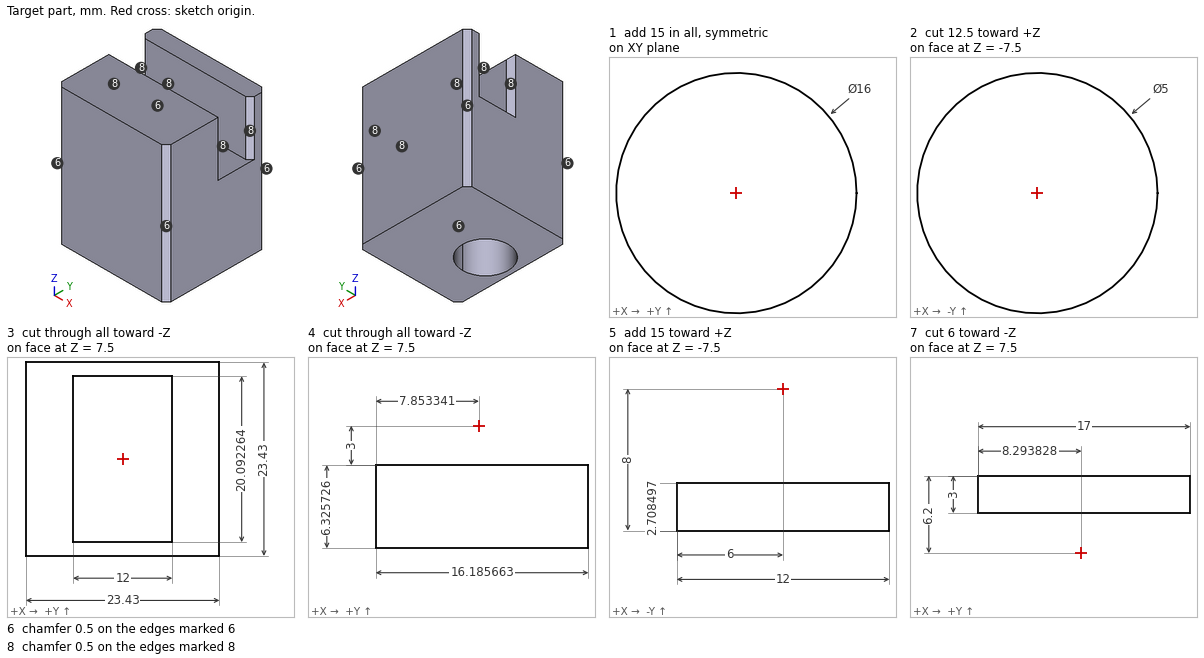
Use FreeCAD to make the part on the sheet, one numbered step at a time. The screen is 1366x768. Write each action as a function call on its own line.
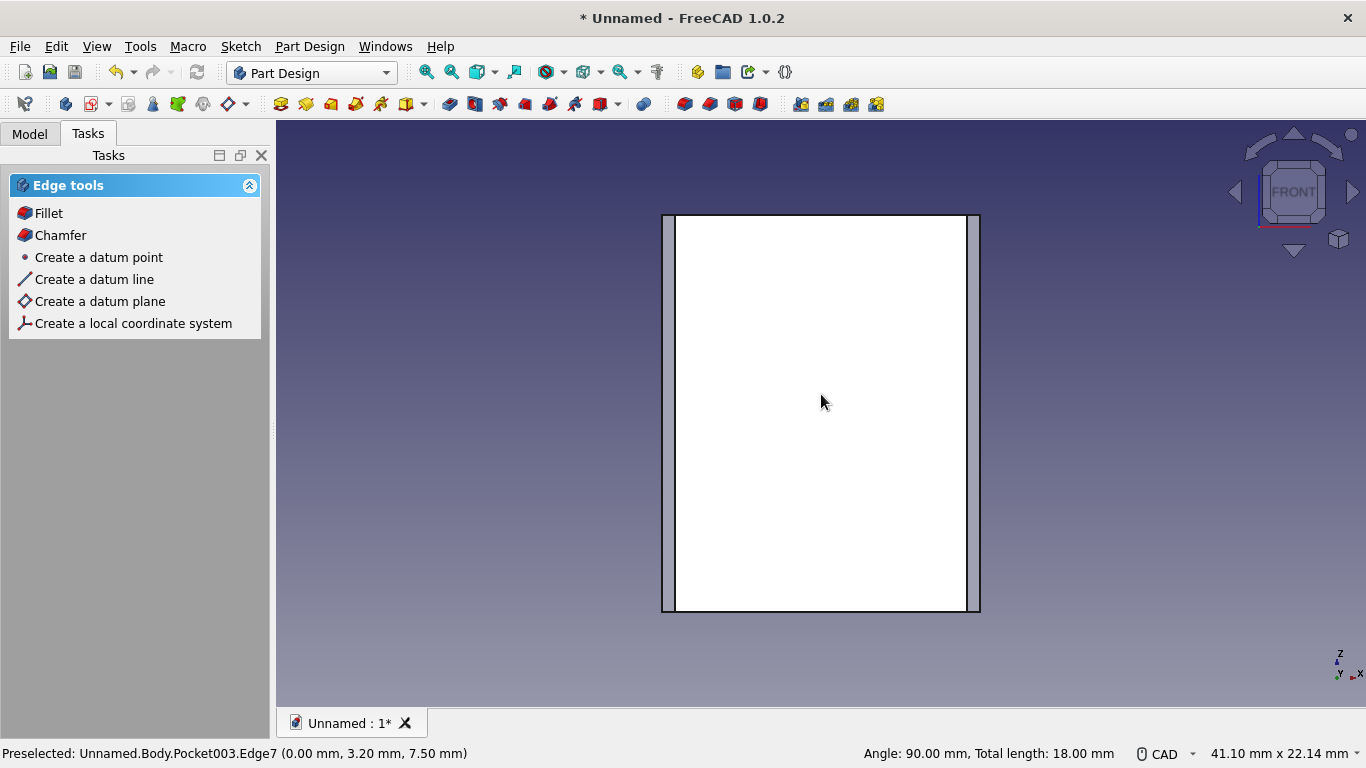
key(3)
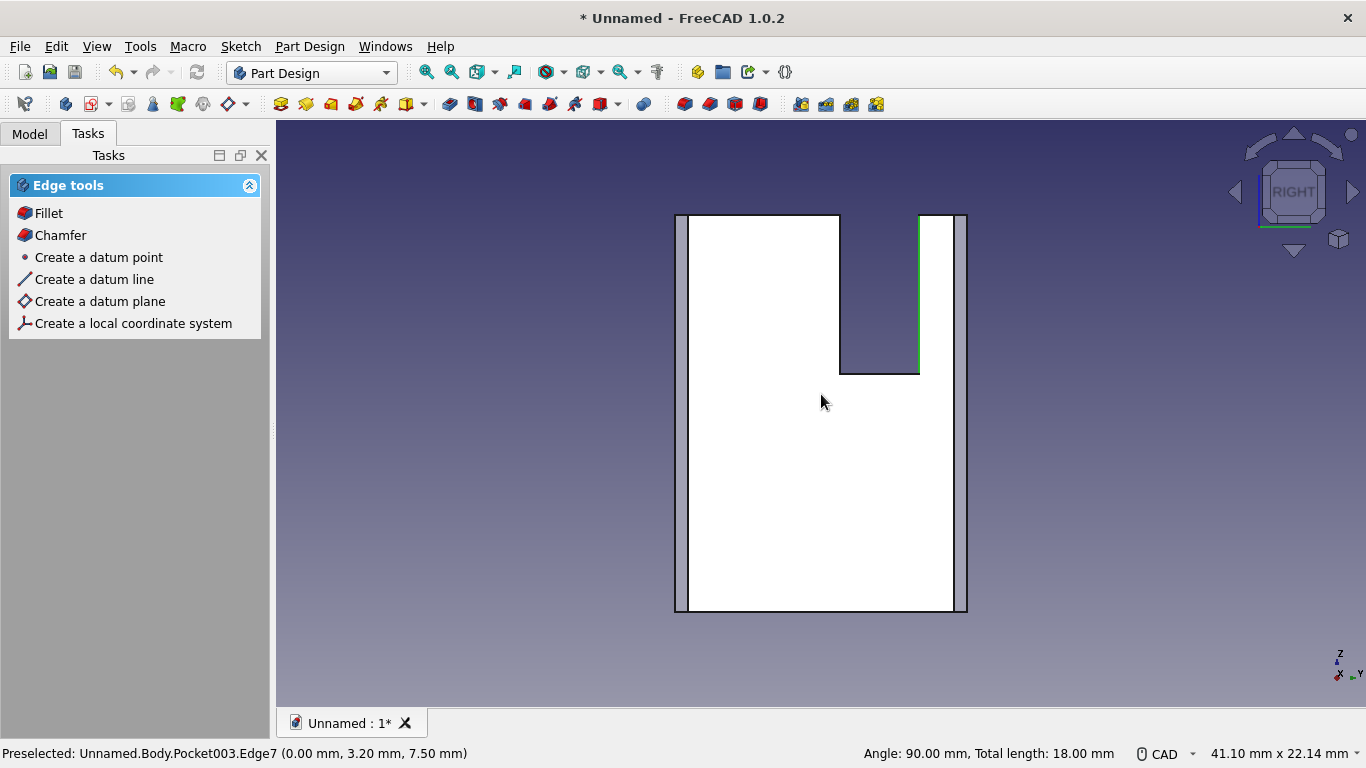
click(840, 293, ctrl)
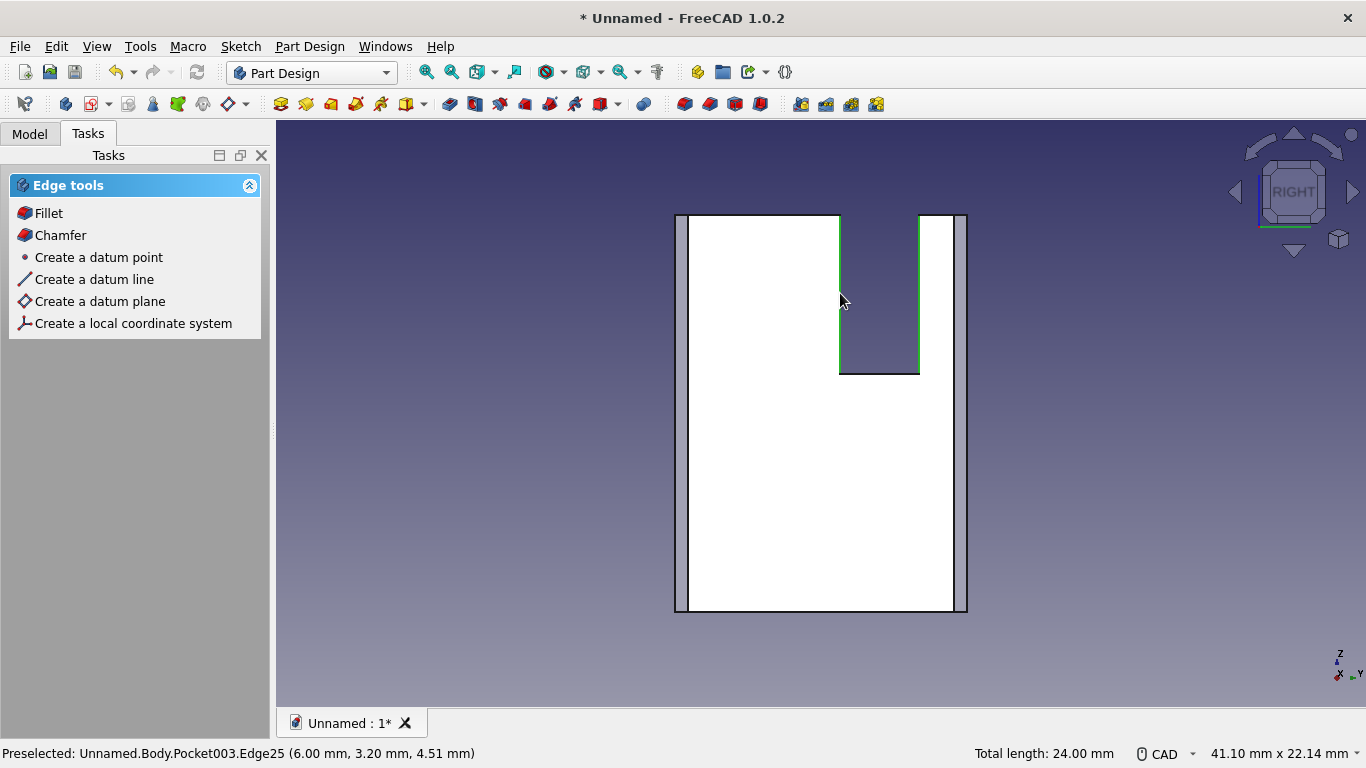
key(5)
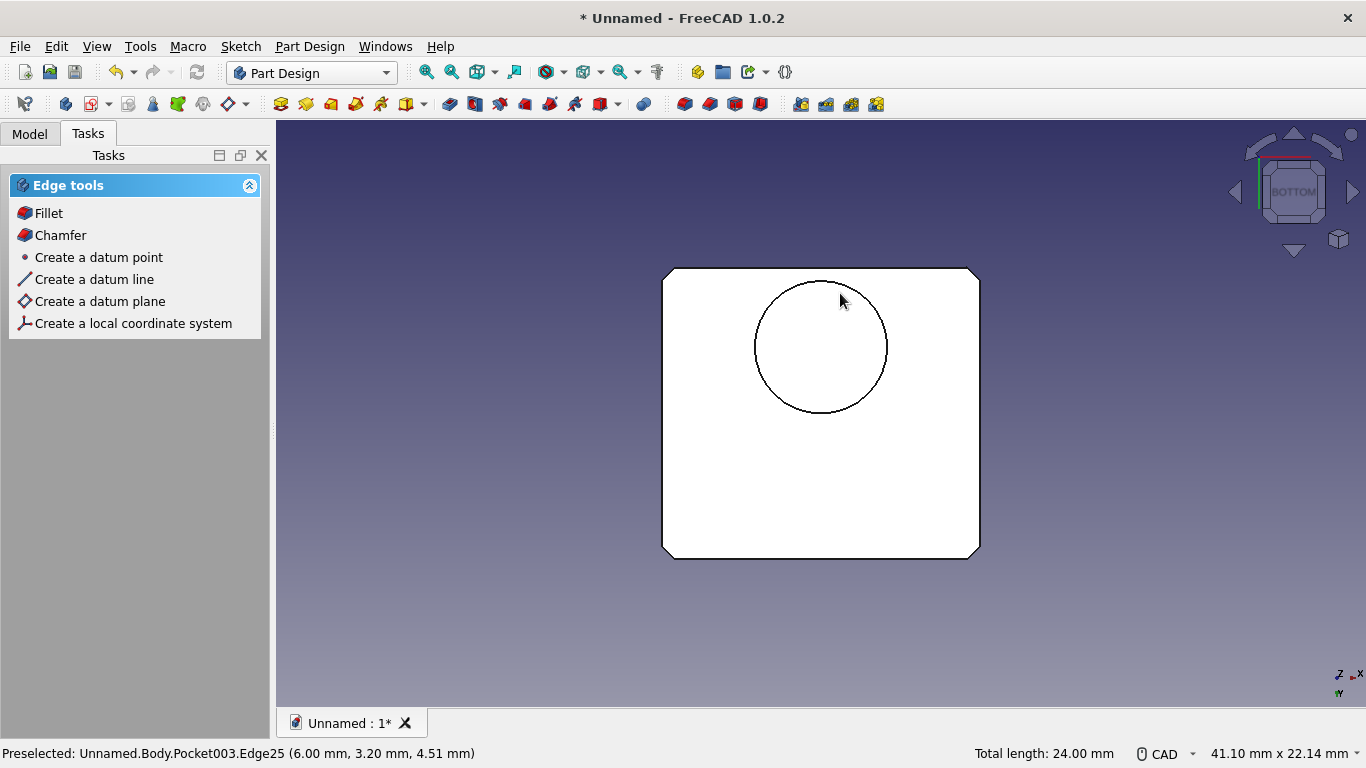
key(4)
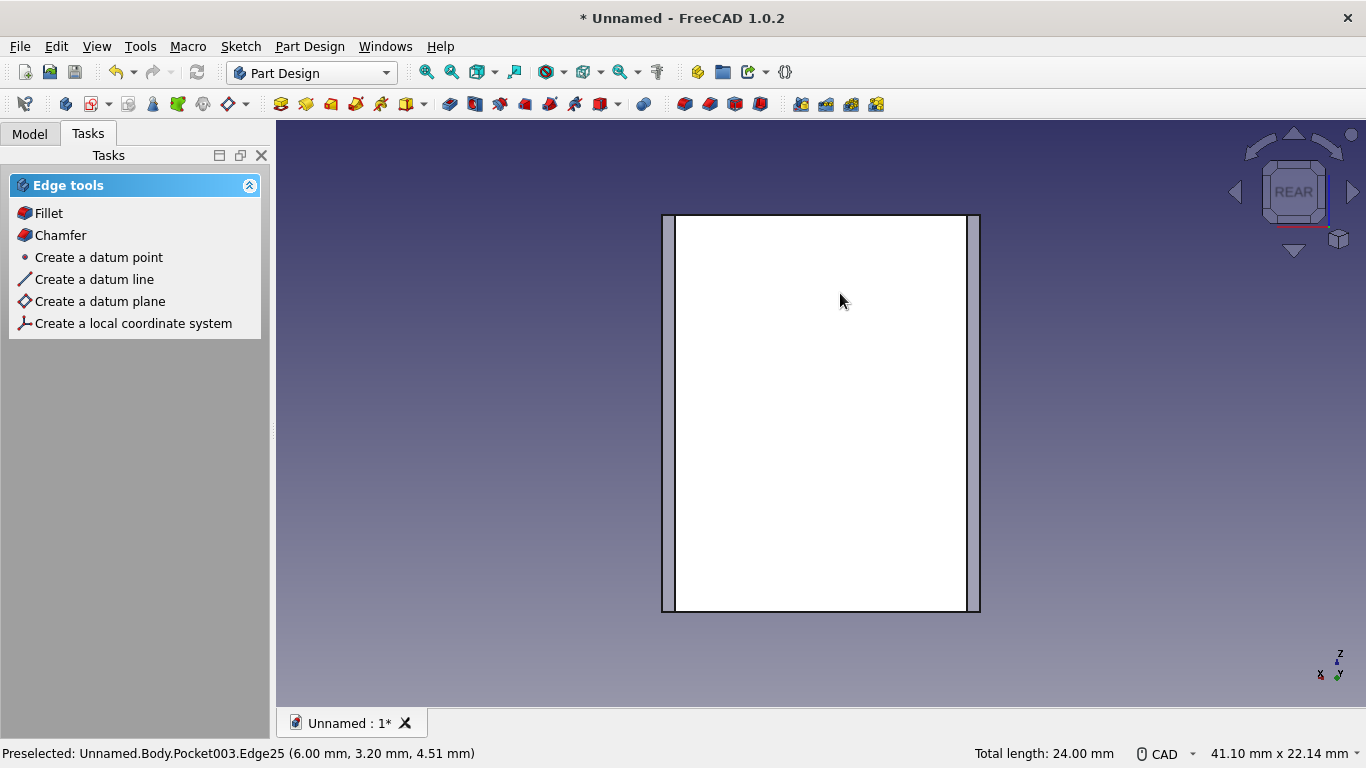
key(6)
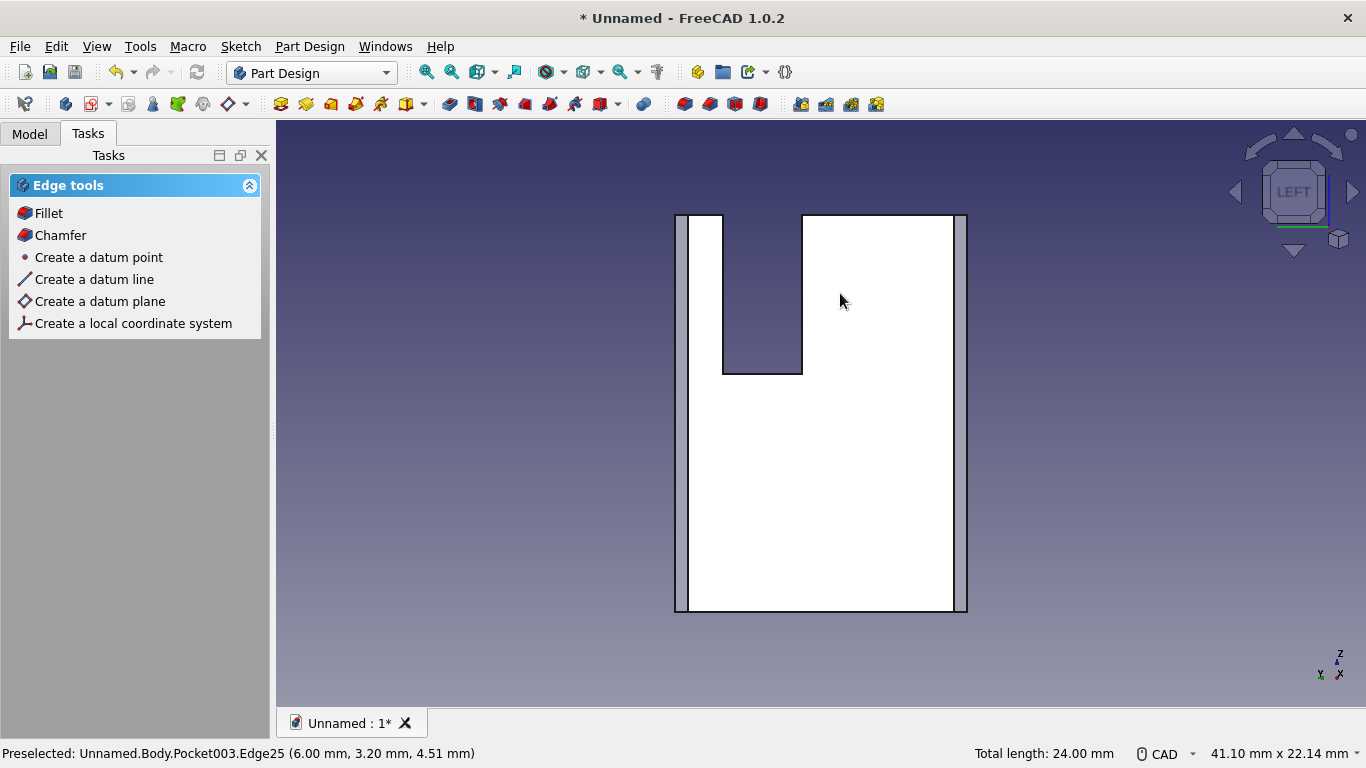
click(723, 293, ctrl)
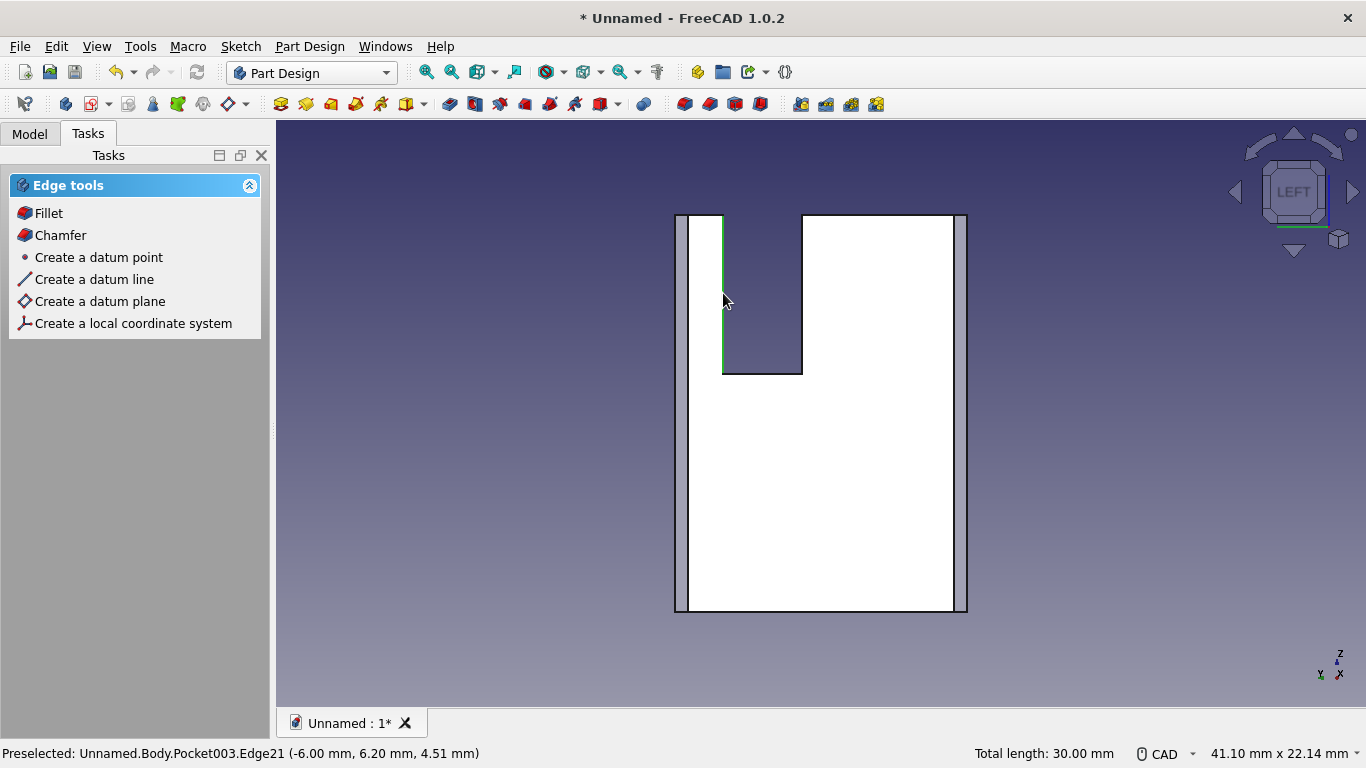
click(802, 293, ctrl)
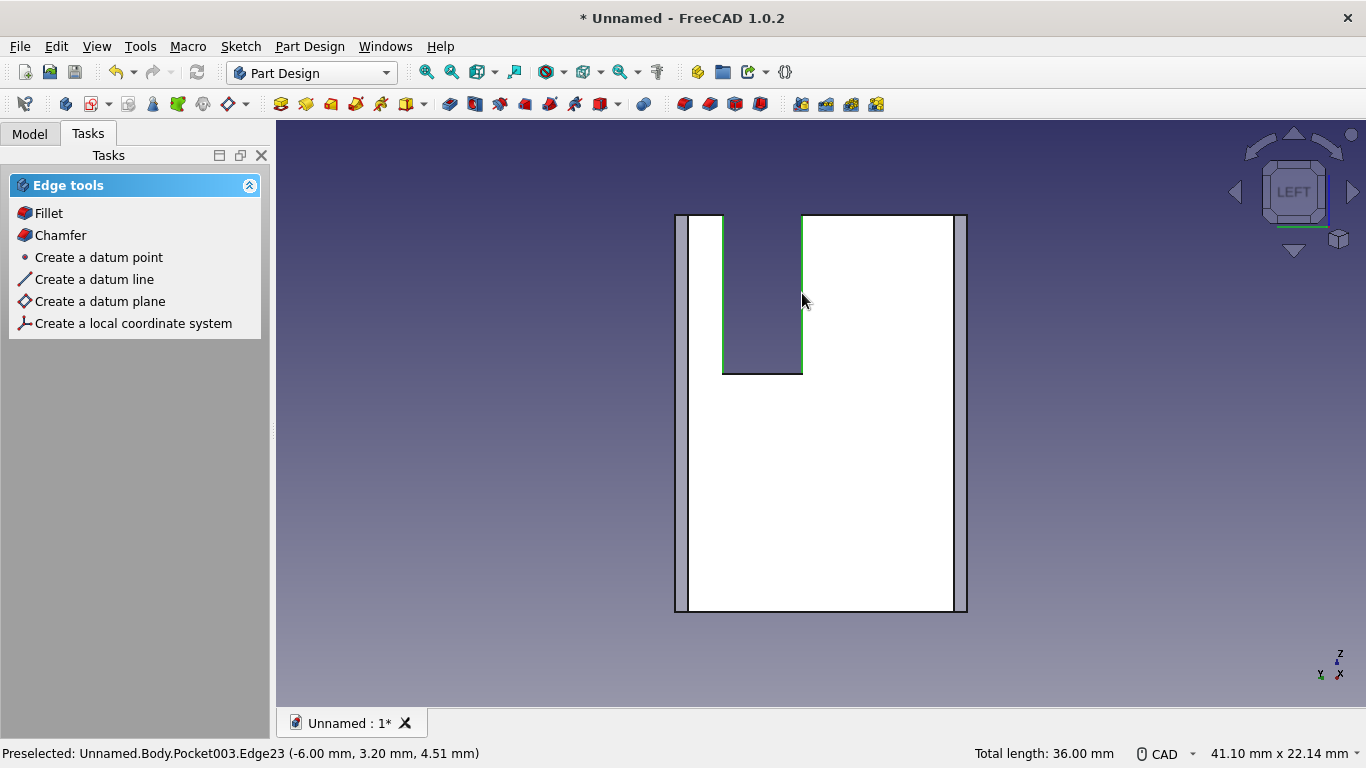
click(710, 104)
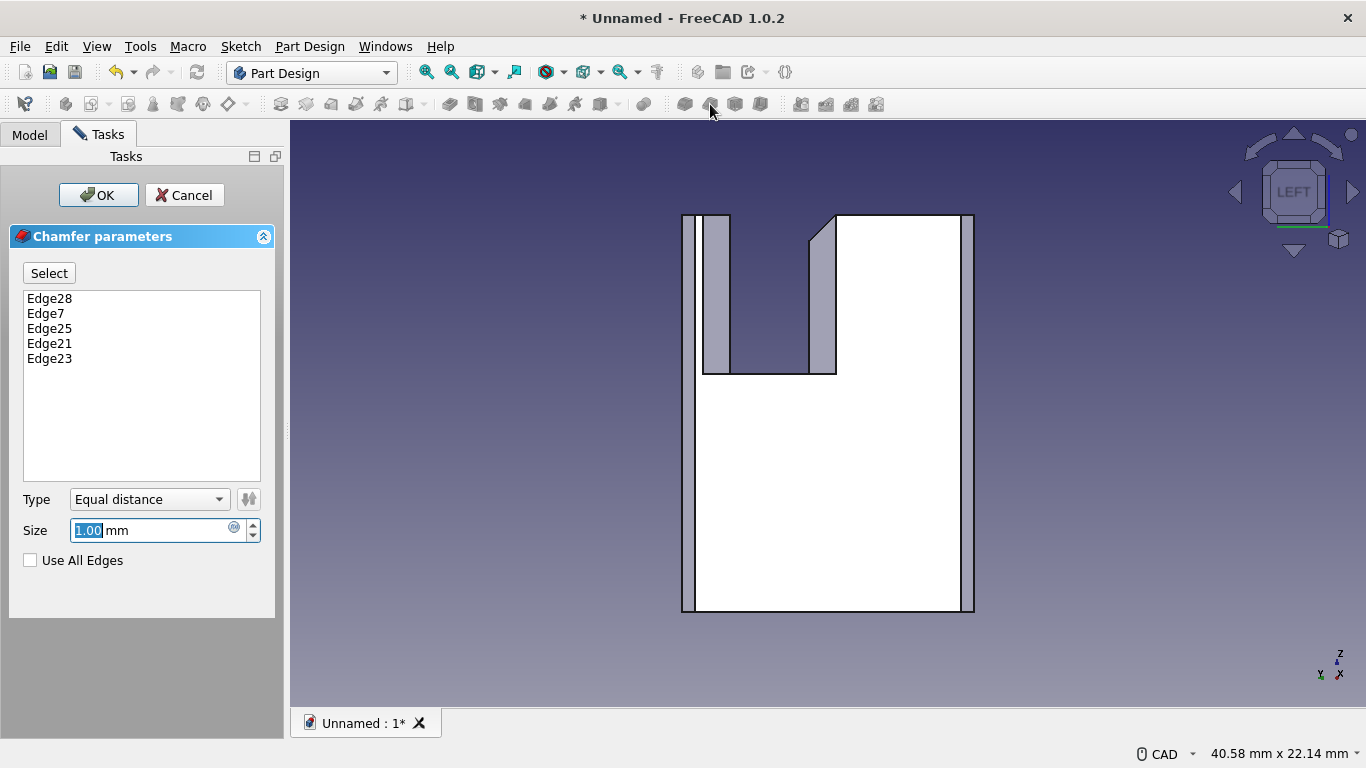
text(0.5)
key(Tab)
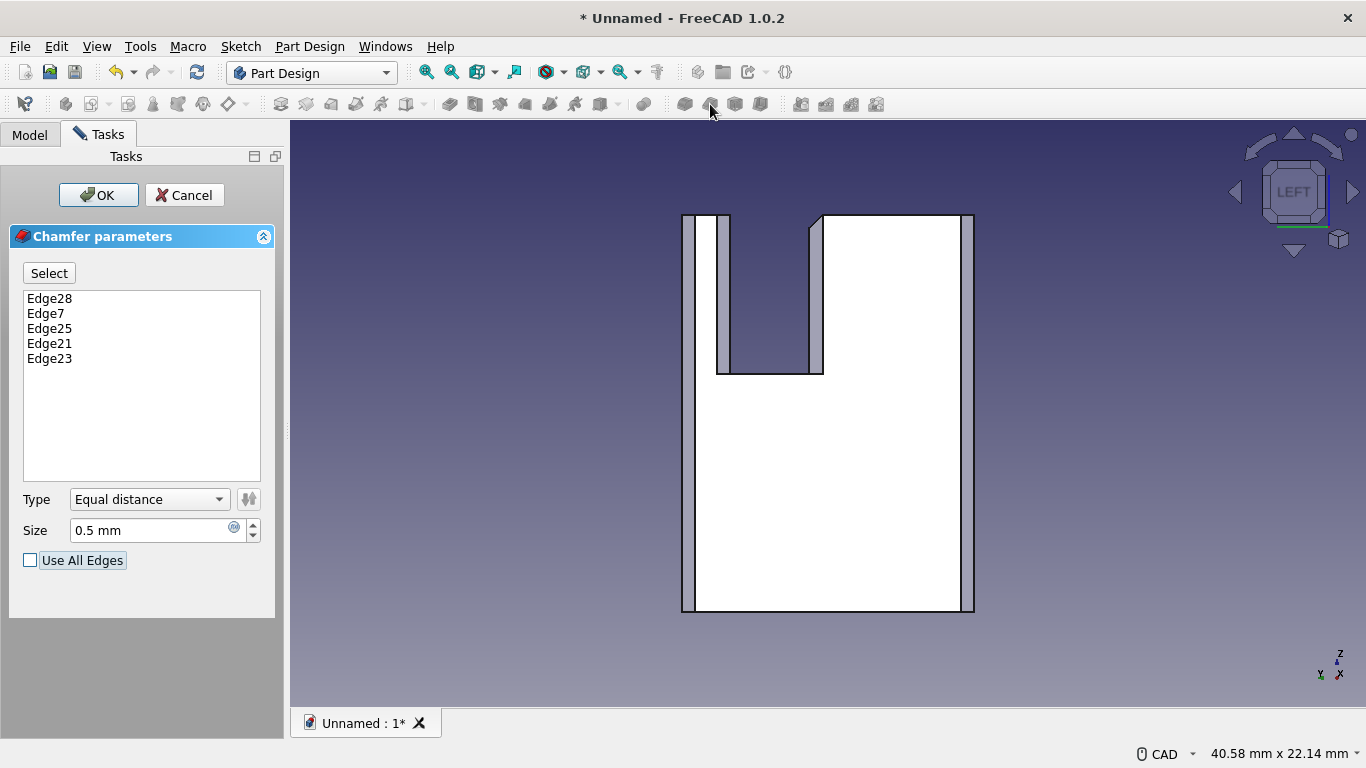
click(99, 195)